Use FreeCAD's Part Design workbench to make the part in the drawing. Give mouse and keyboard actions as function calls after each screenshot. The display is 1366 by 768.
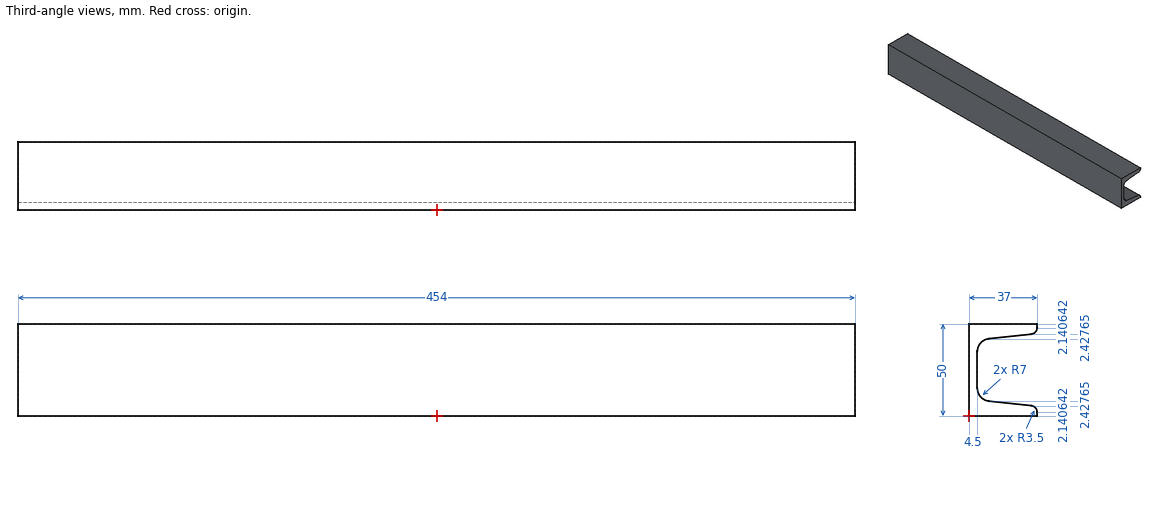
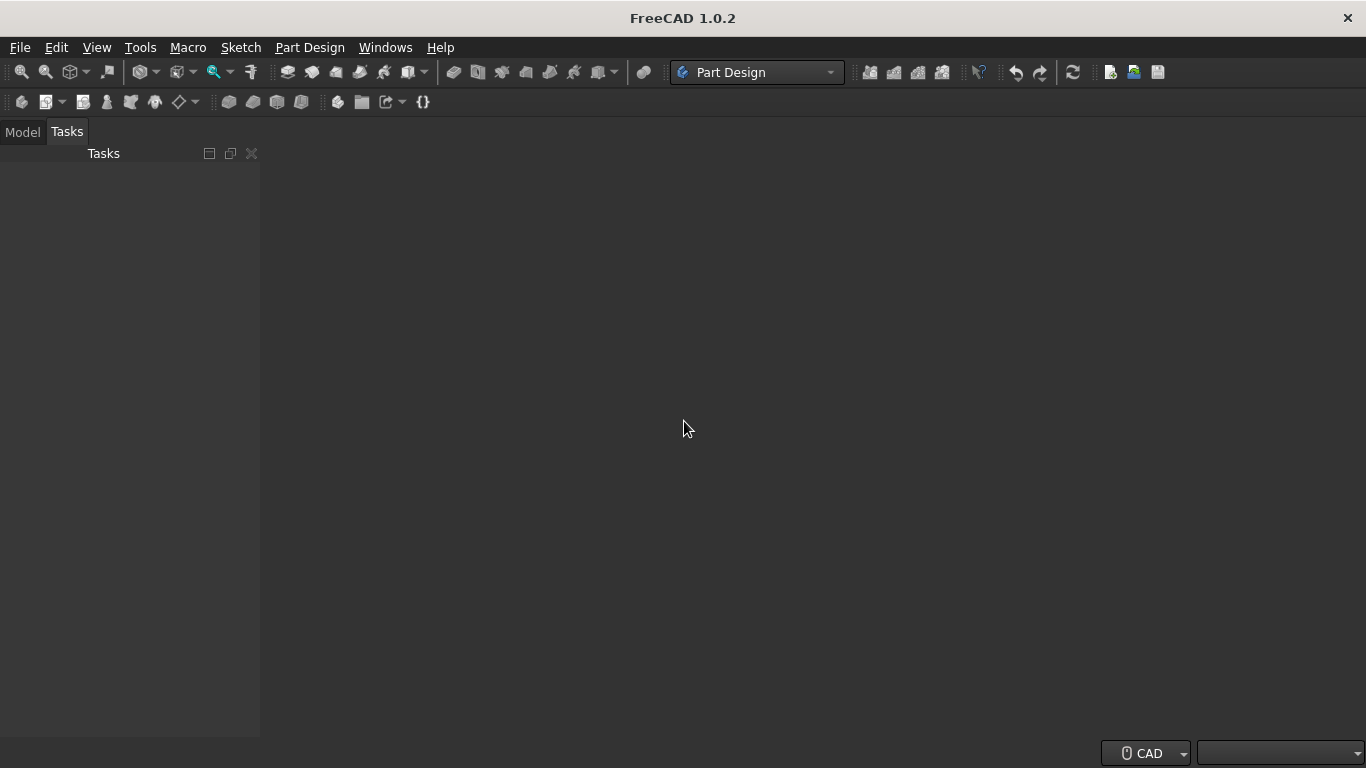
click(1110, 72)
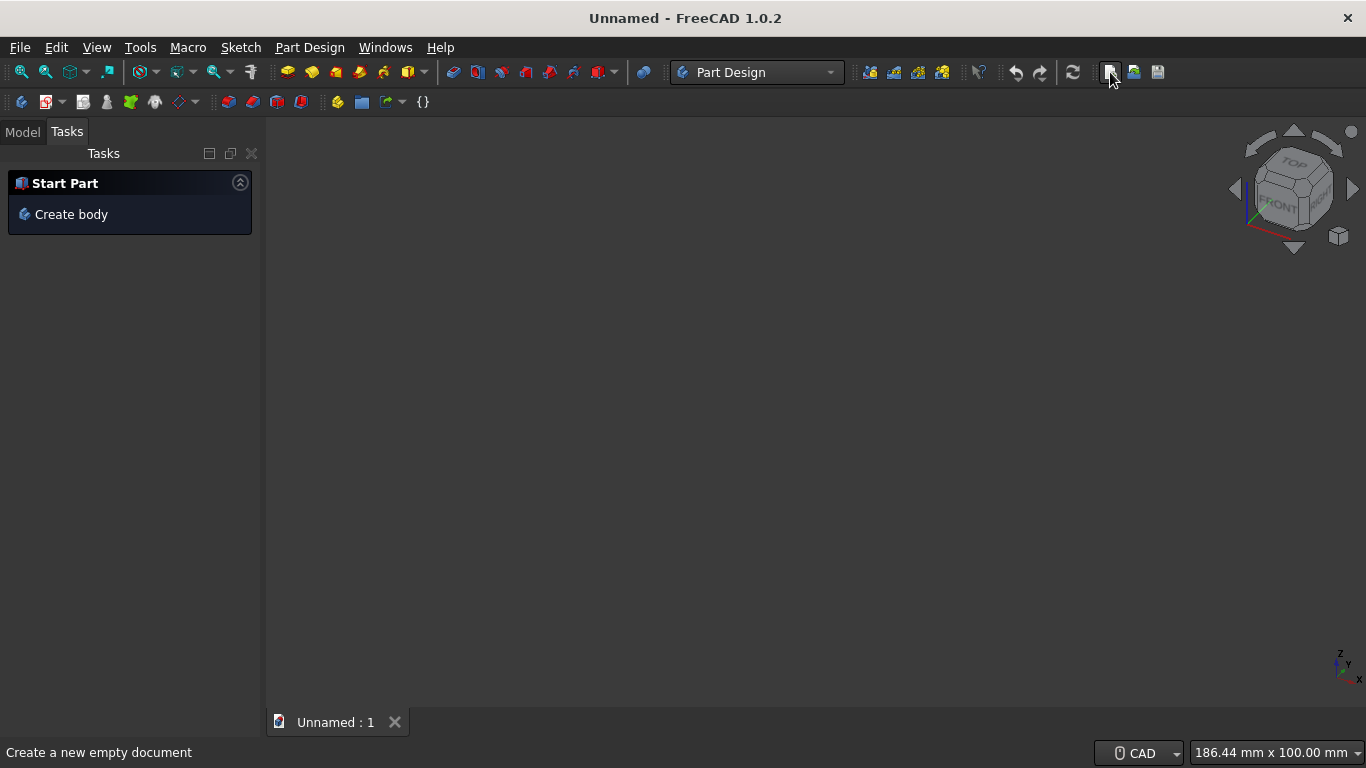
click(22, 102)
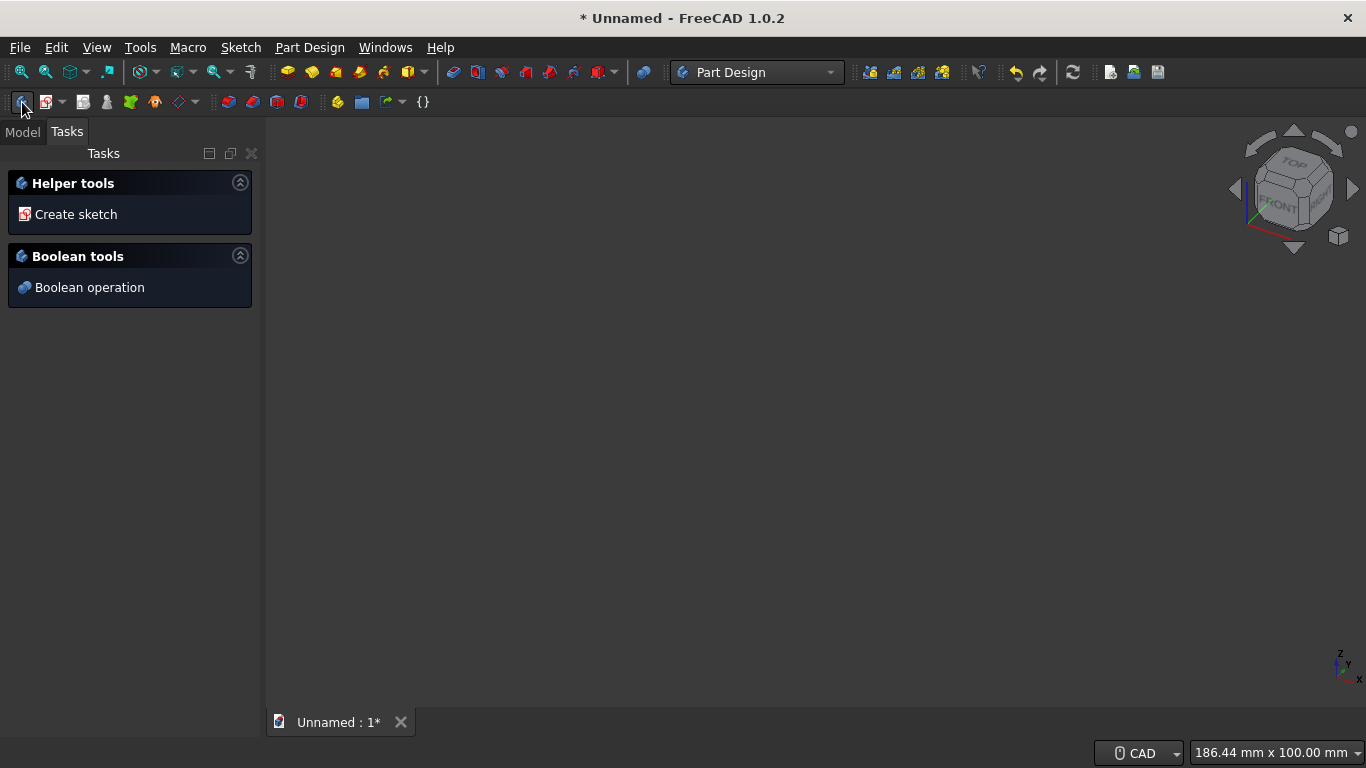
click(23, 131)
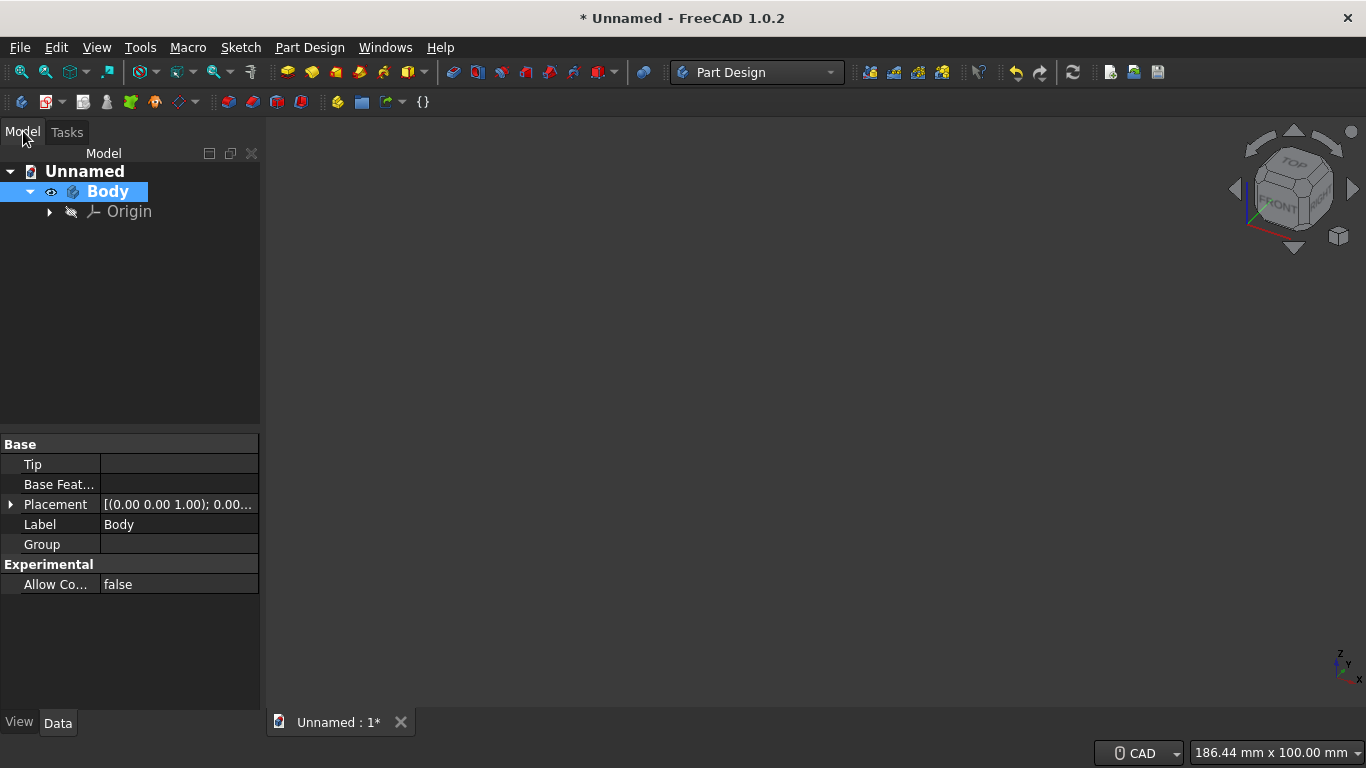
click(50, 212)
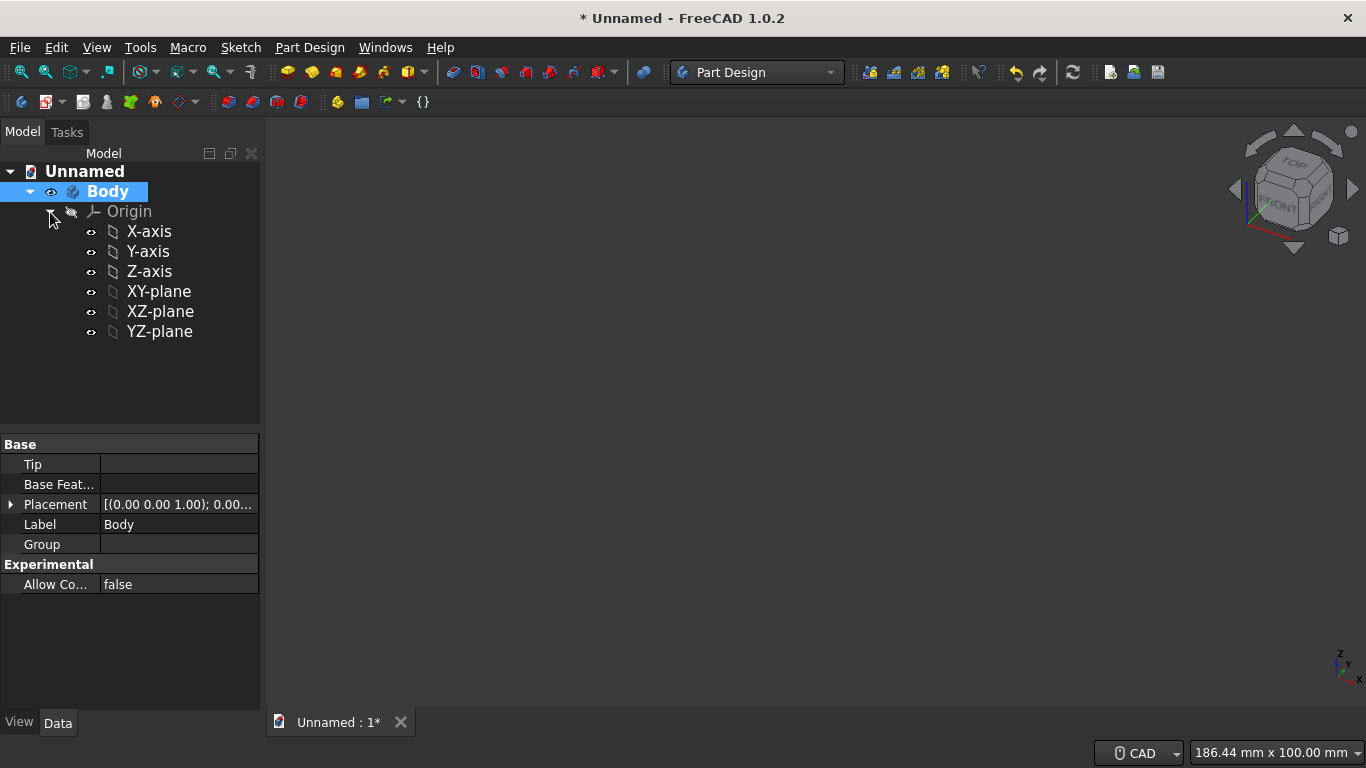
click(136, 332)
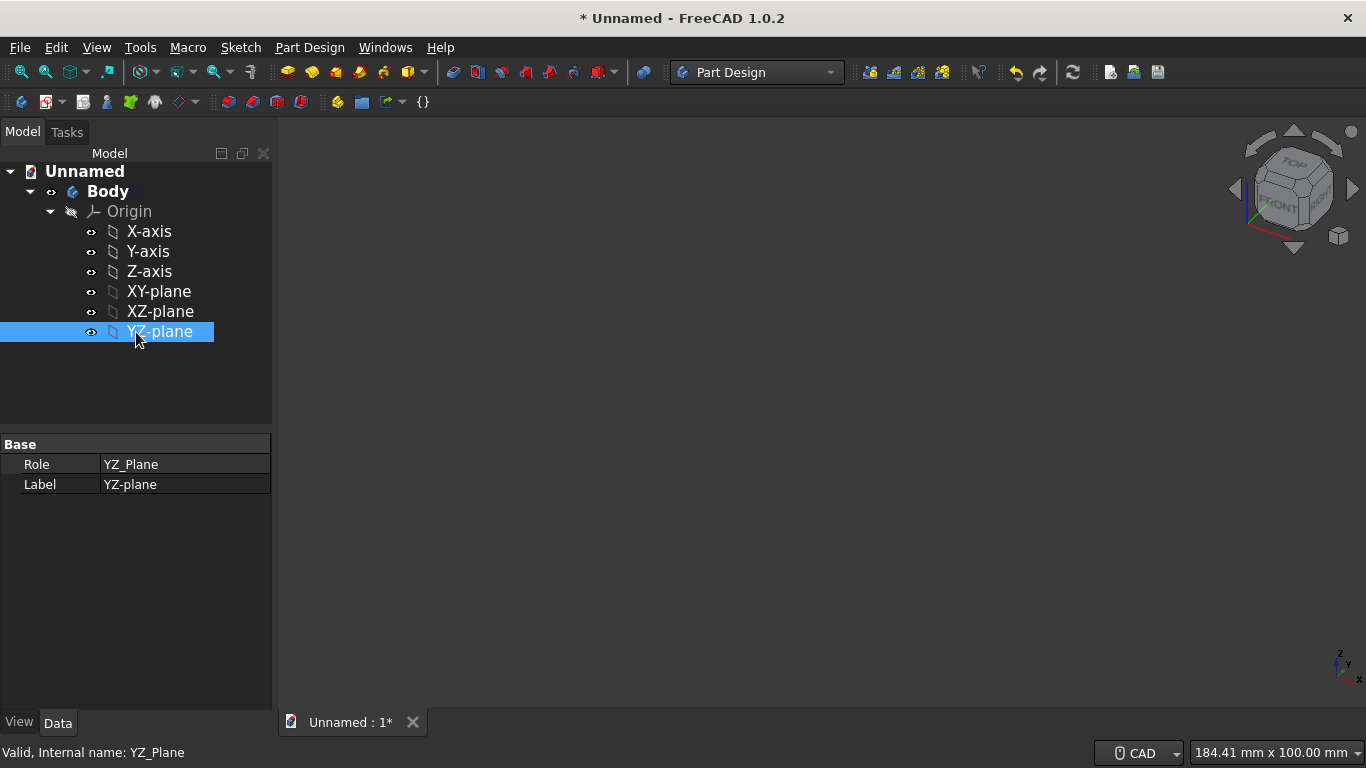
click(180, 102)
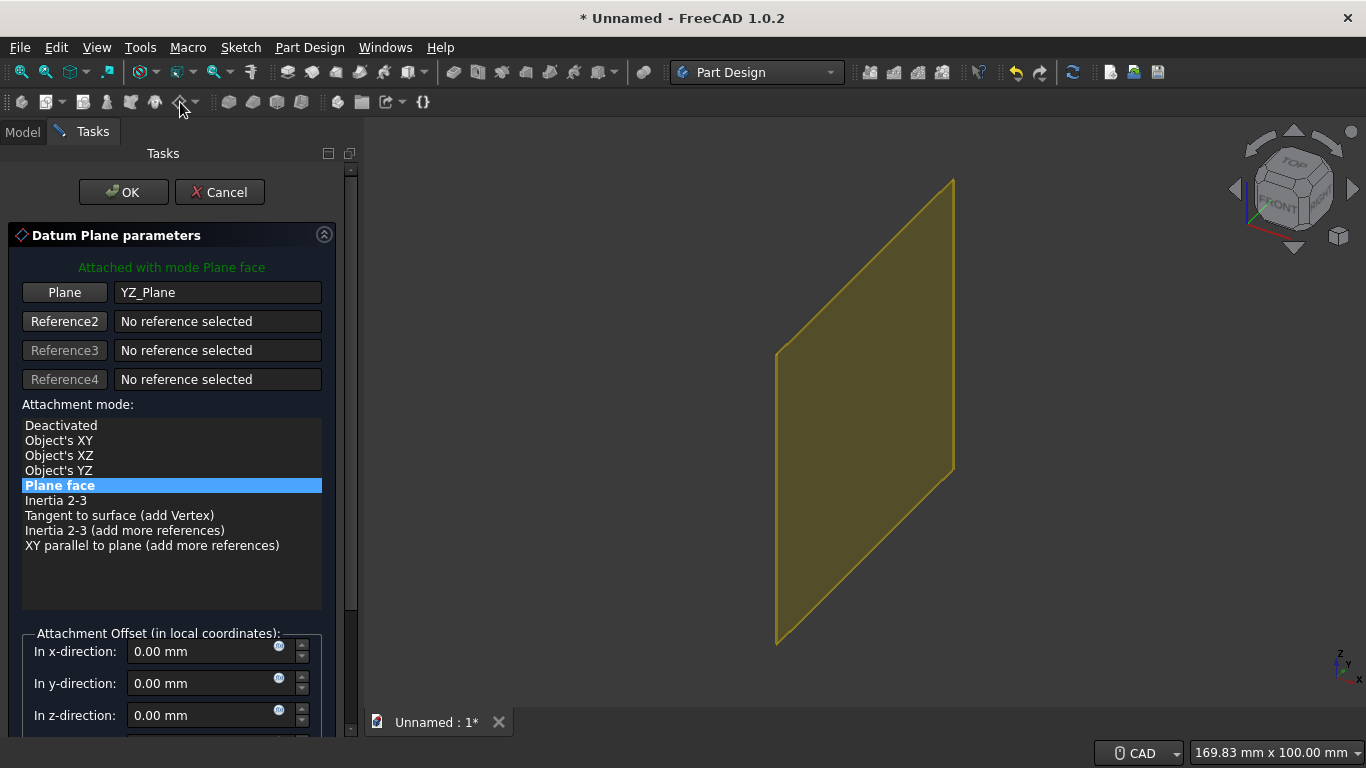
triple_click(210, 715)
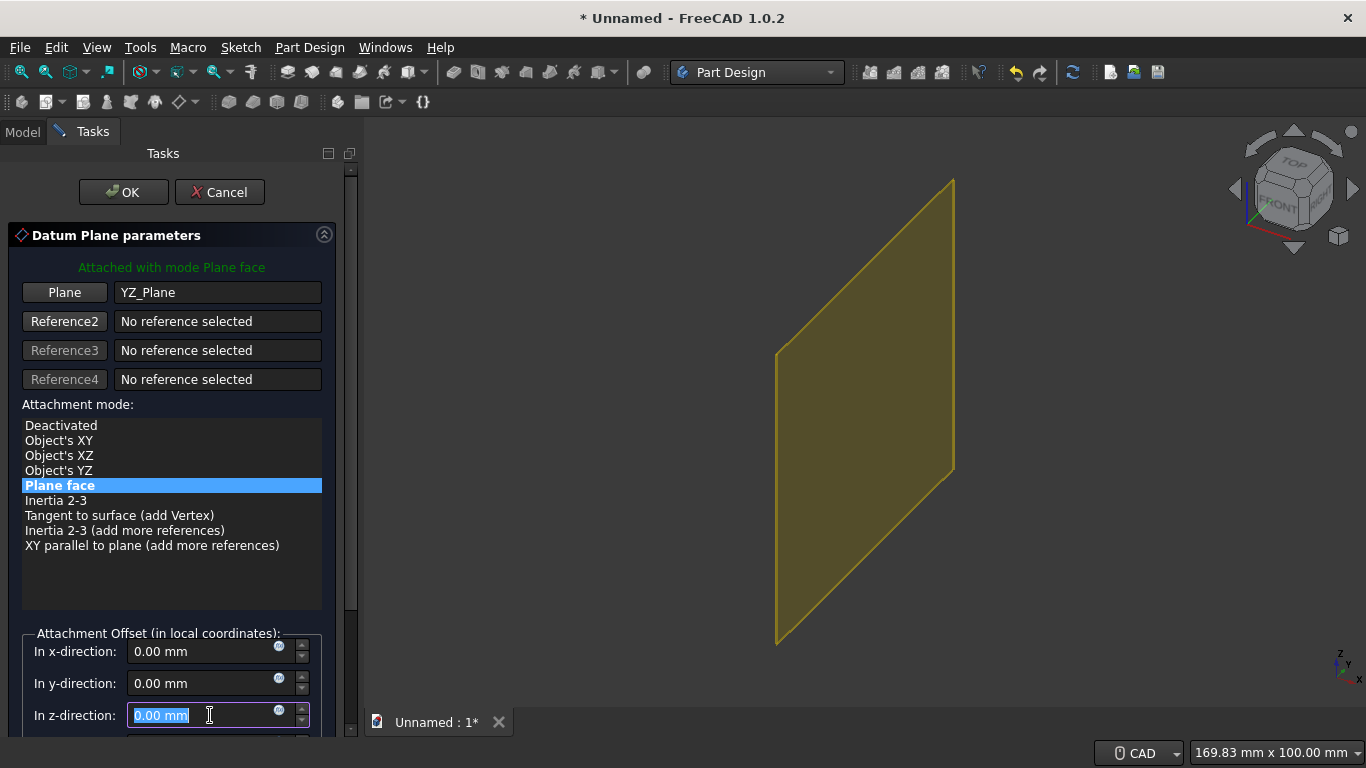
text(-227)
key(Tab)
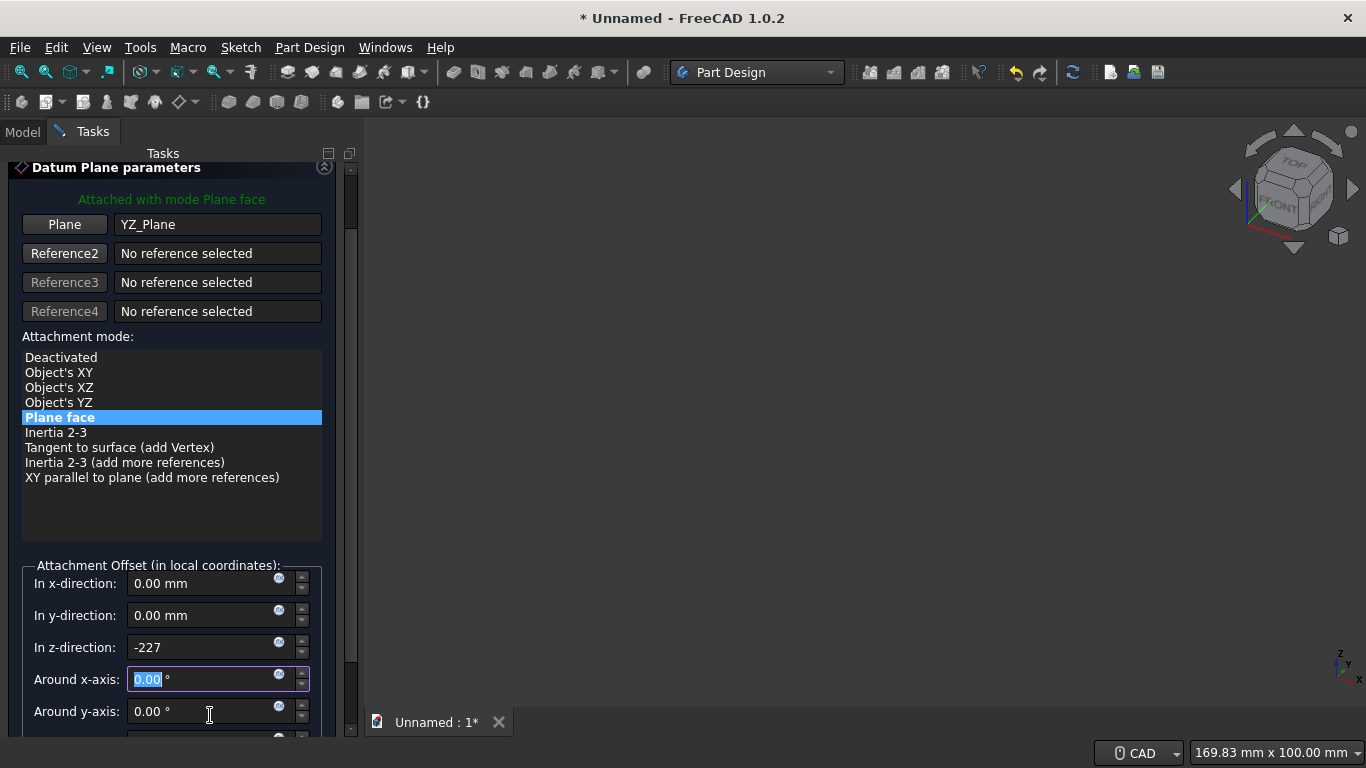
scroll(351, 450, up, 2)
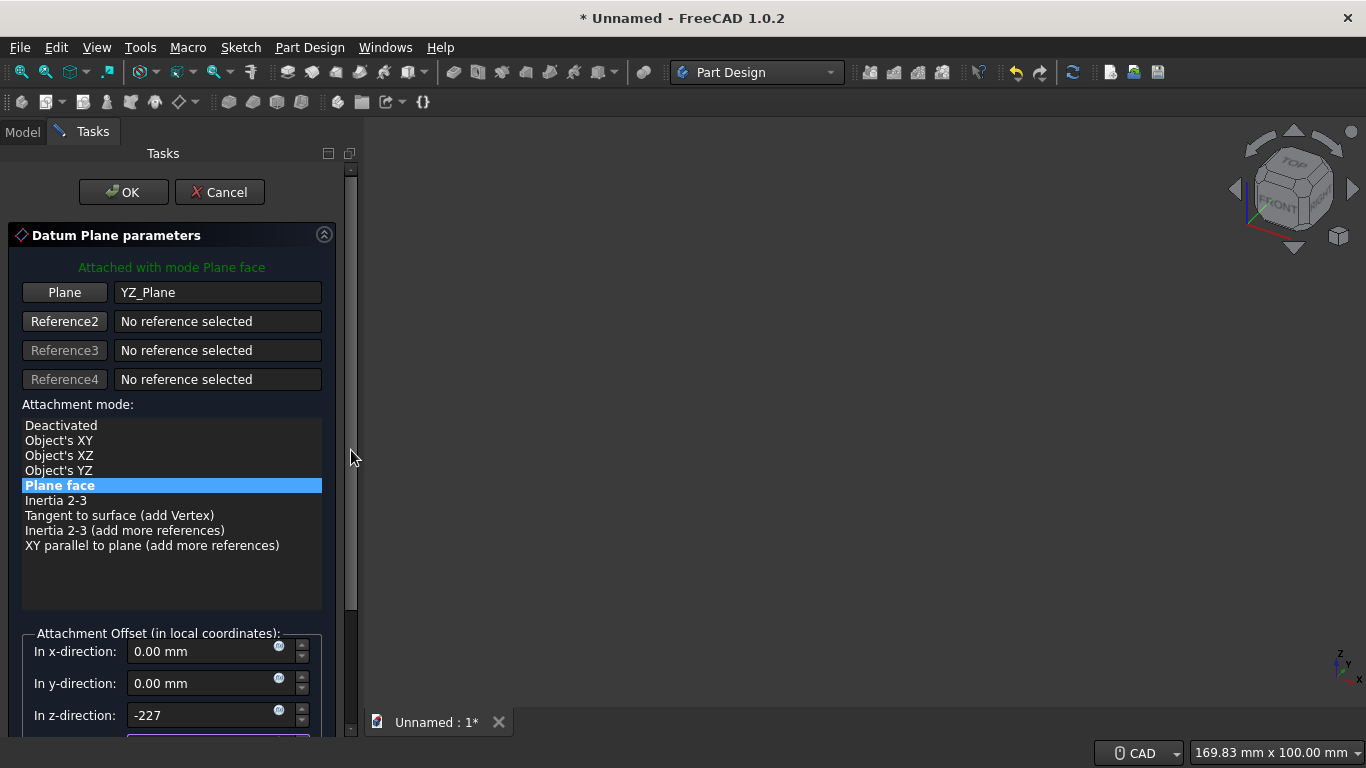
click(124, 192)